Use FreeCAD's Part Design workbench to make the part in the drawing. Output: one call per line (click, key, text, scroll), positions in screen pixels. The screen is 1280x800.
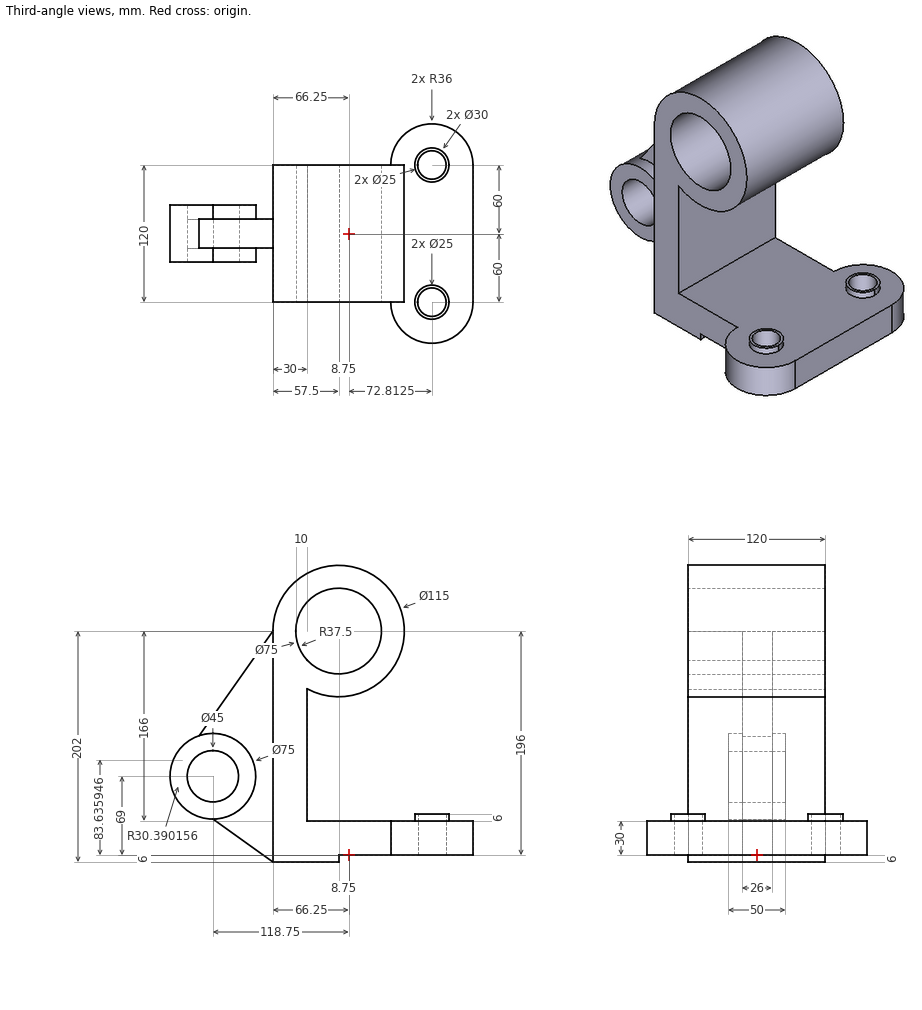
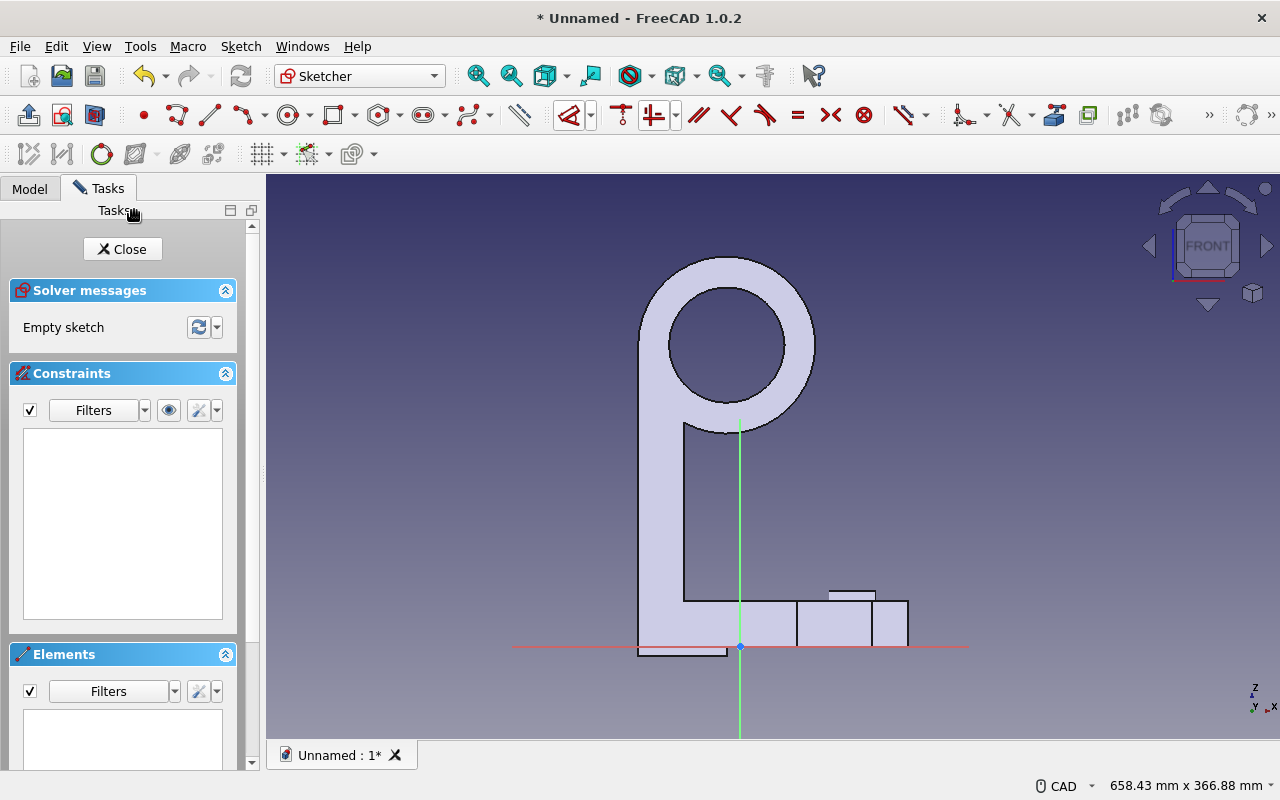
click(516, 518)
click(638, 345)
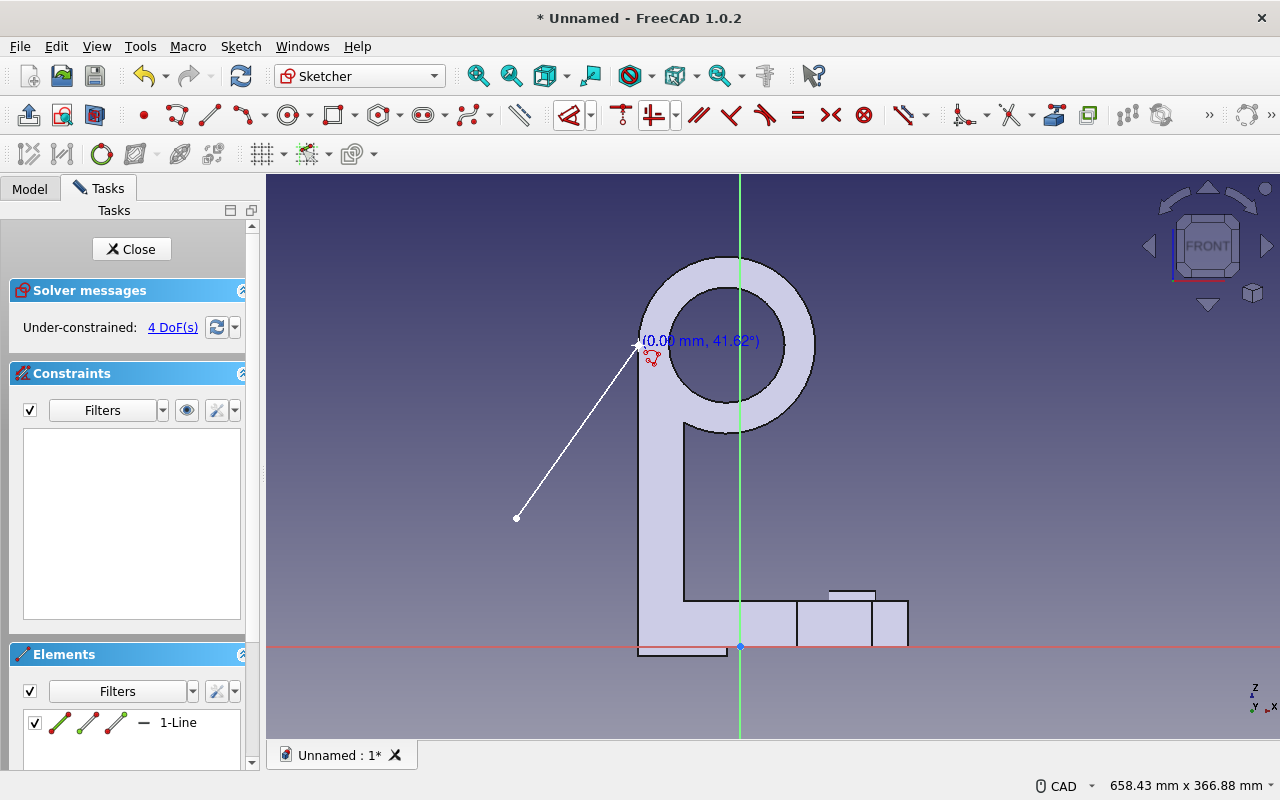
scroll(638, 656, up, 3)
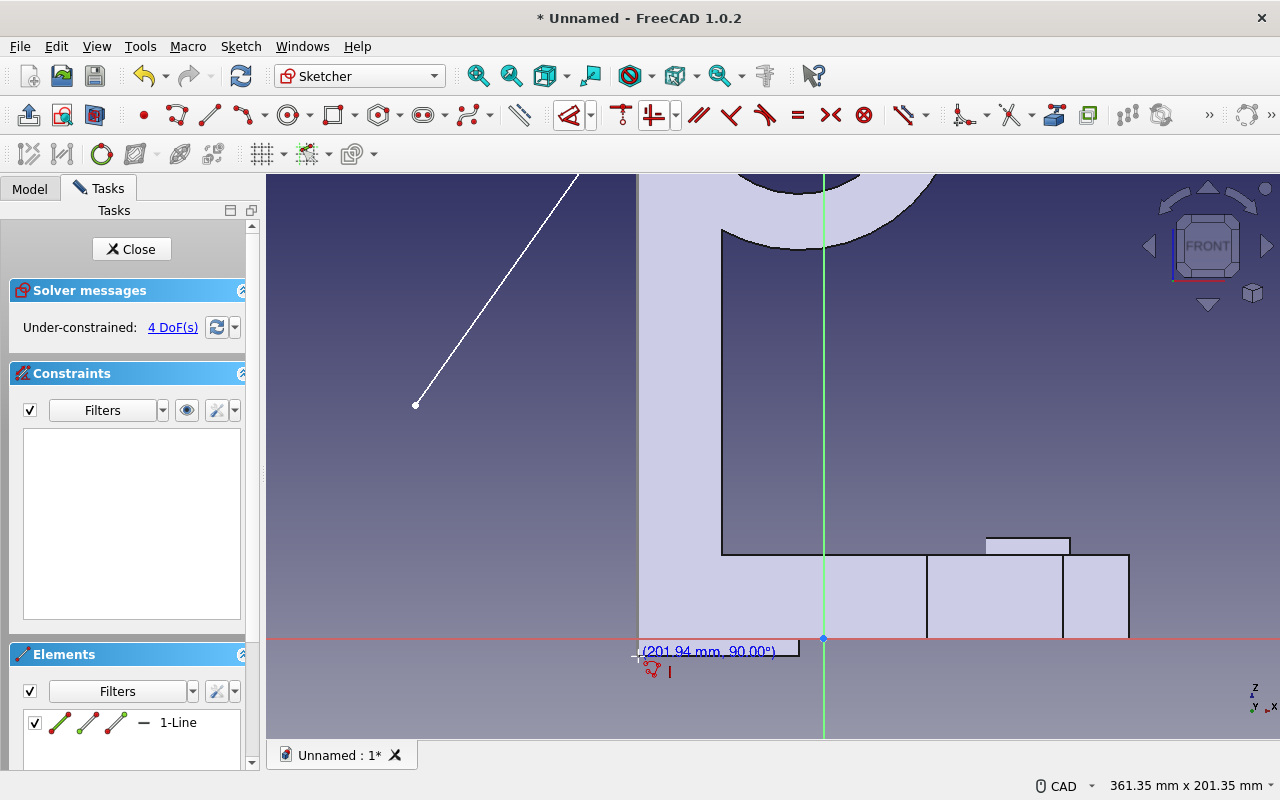
click(638, 656)
click(441, 514)
right_click(441, 514)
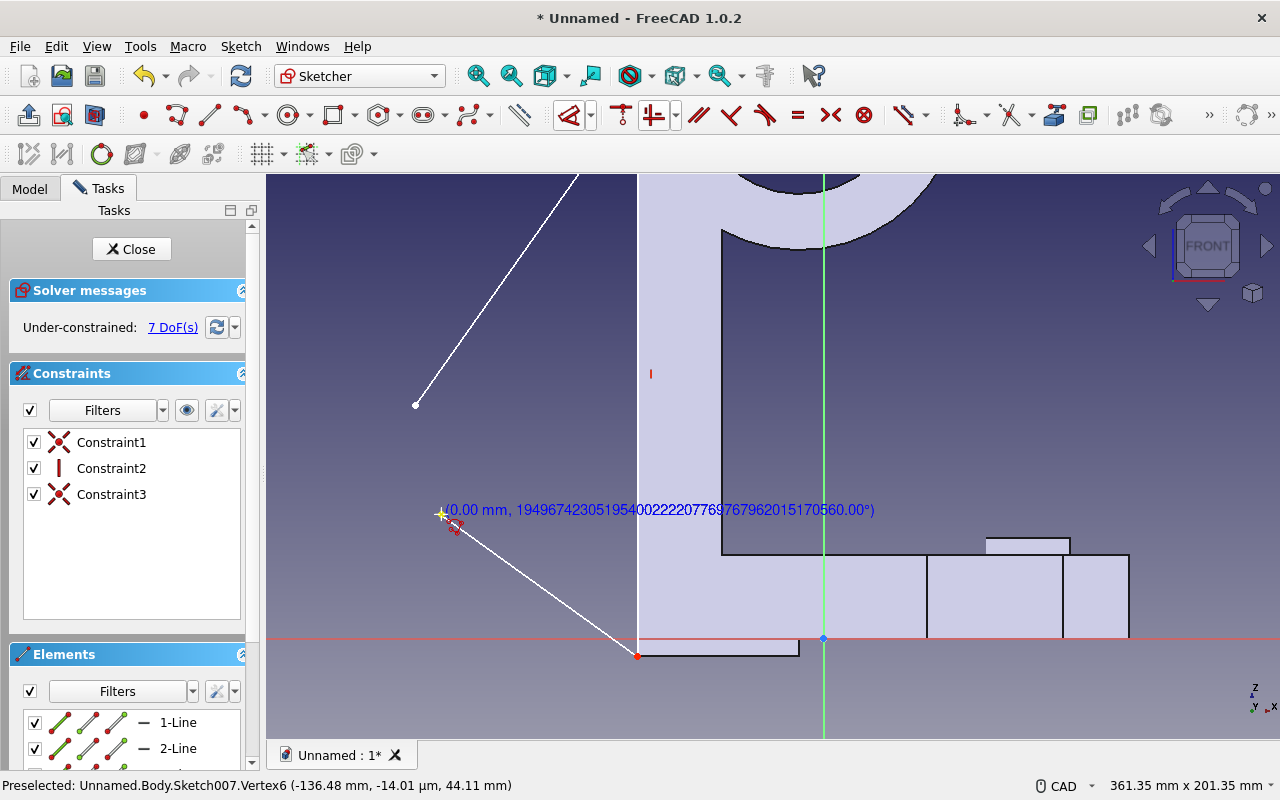
key(g)
key(3)
key(a)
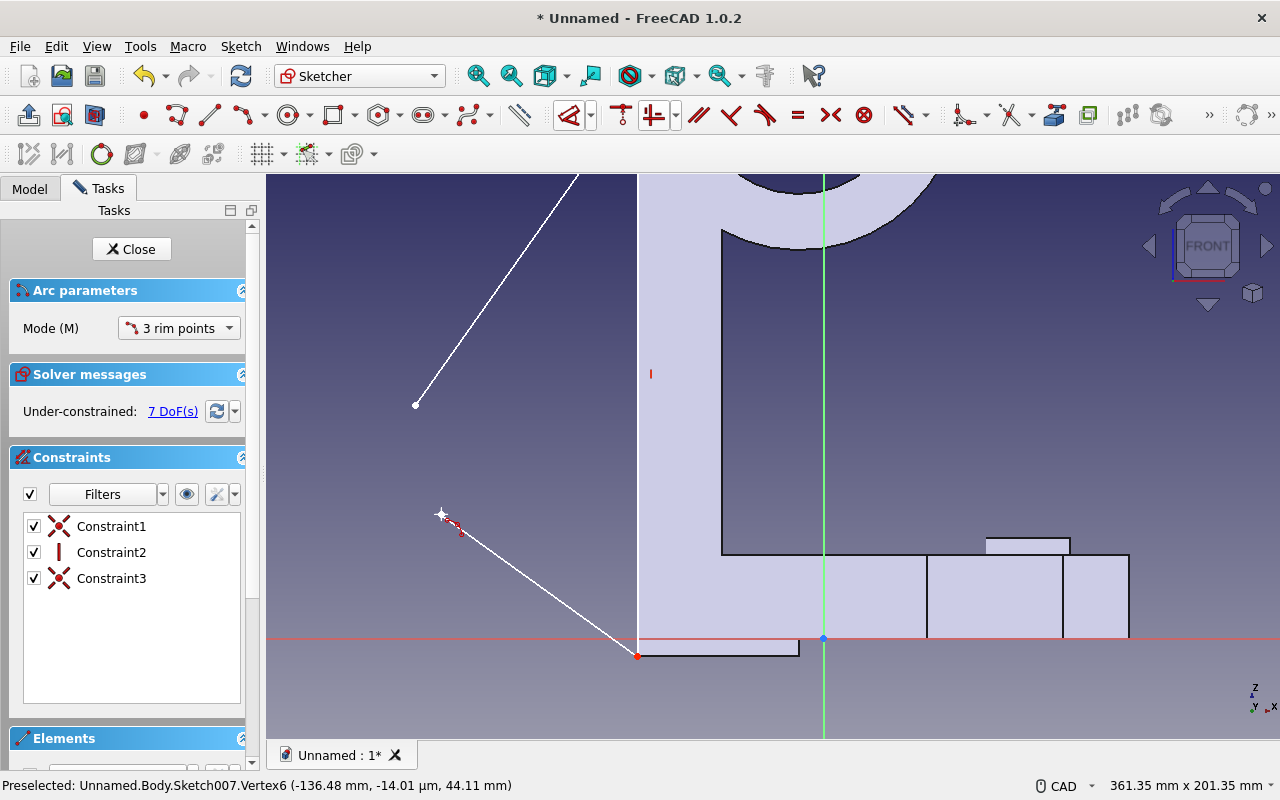
click(441, 515)
click(415, 406)
click(408, 464)
key(Escape)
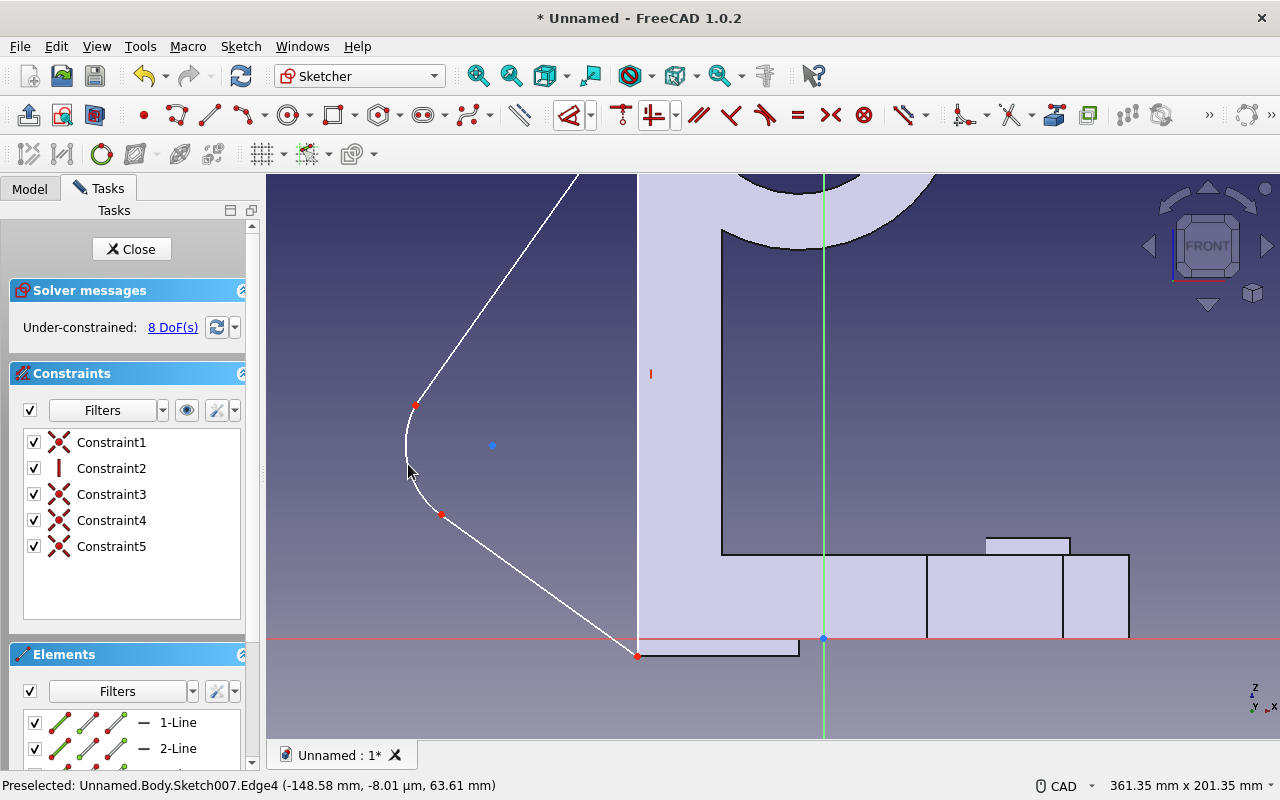
click(579, 614)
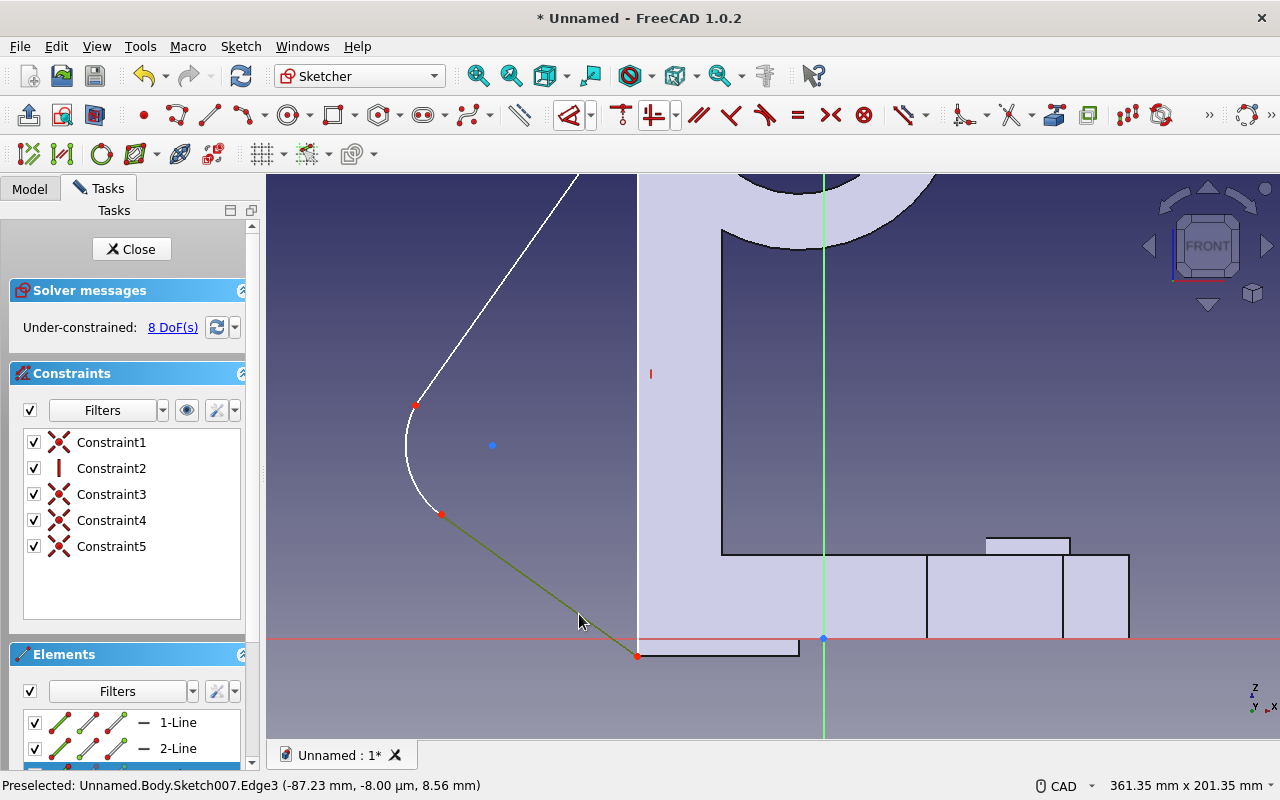
click(406, 441)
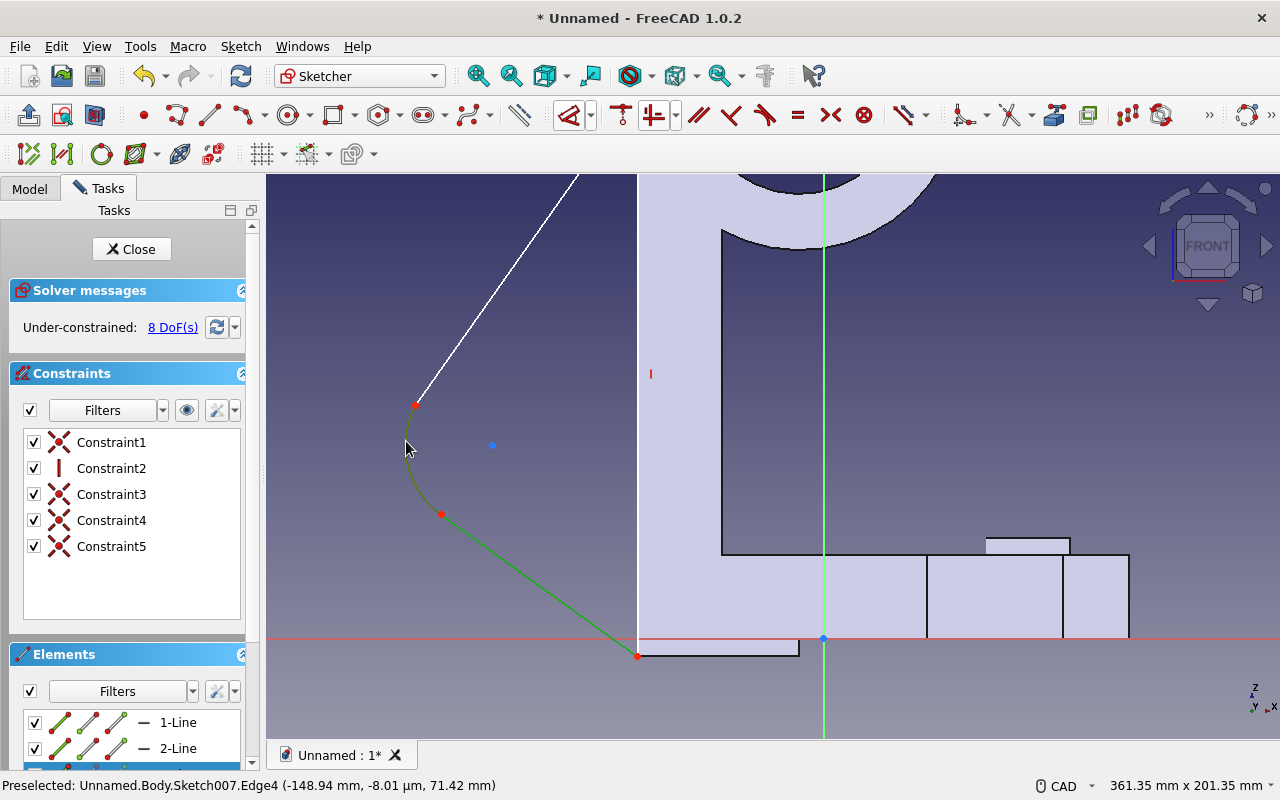
key(t)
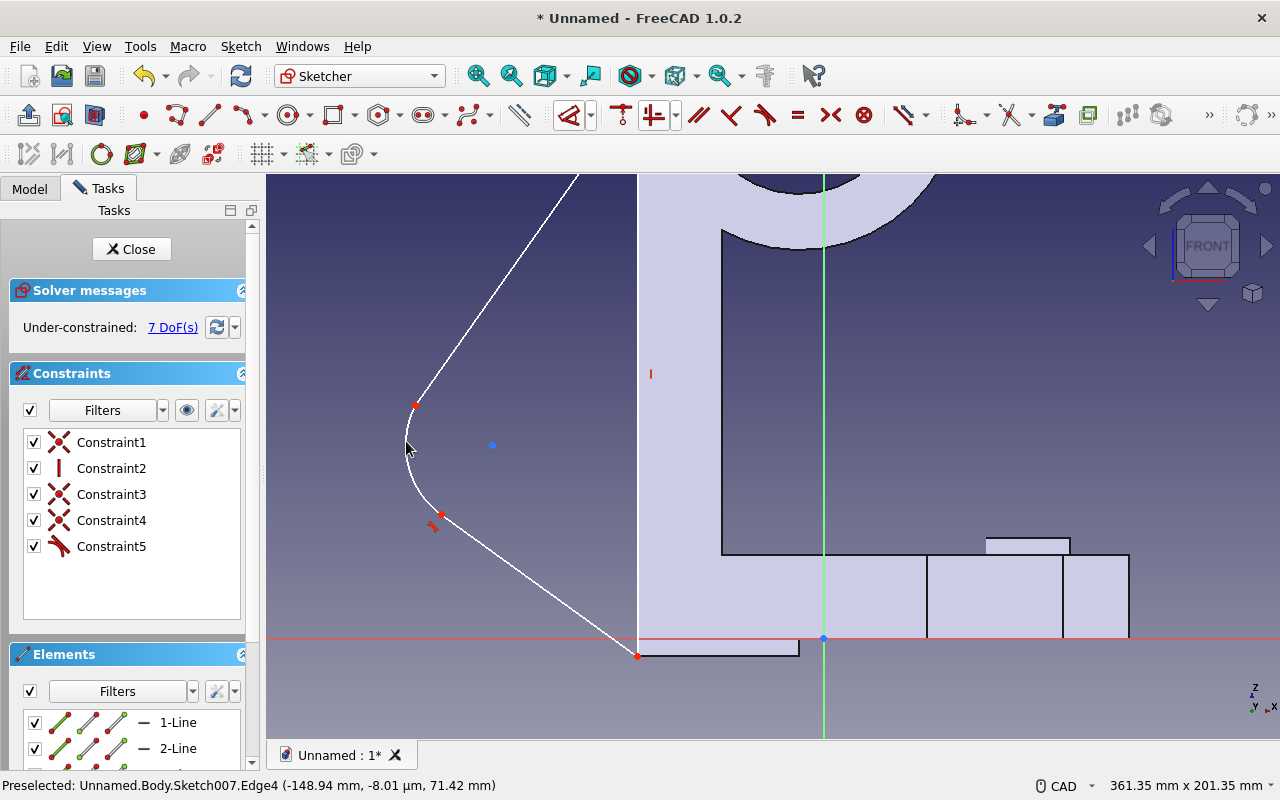
click(406, 441)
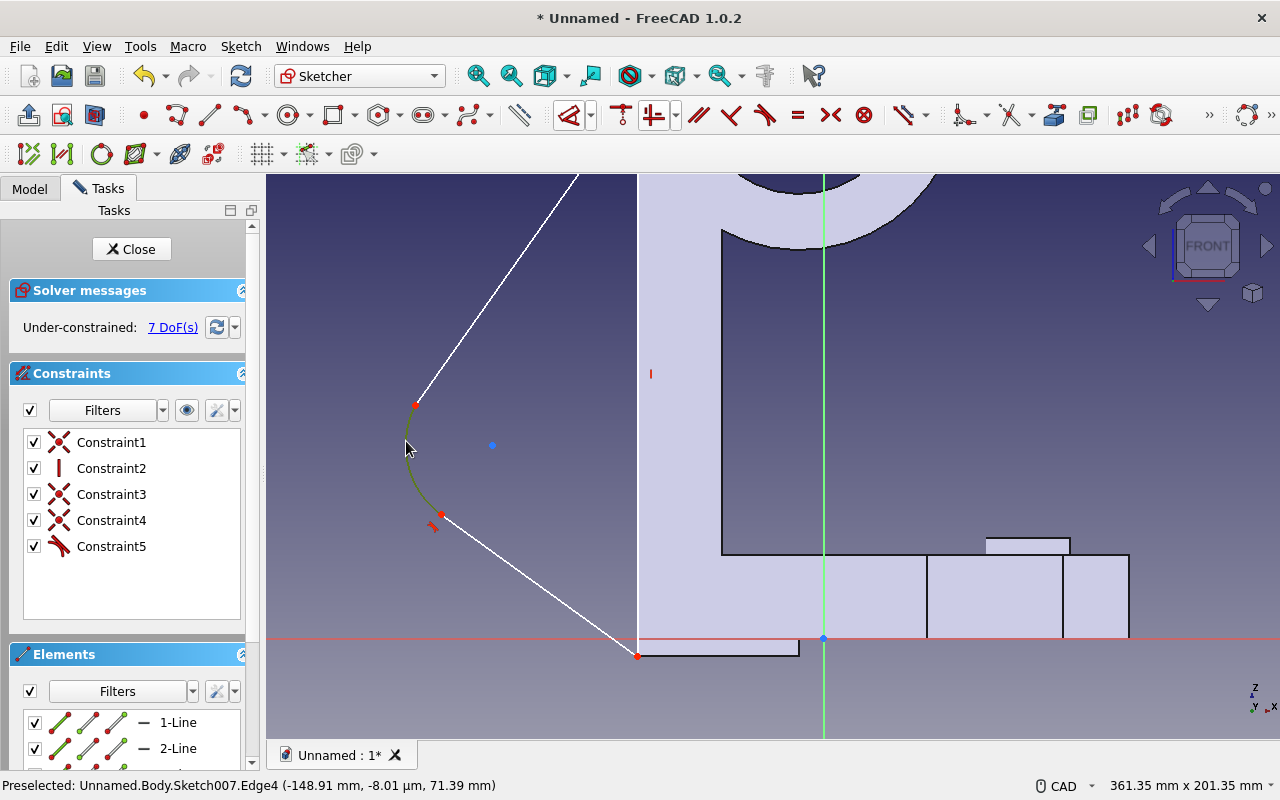
click(590, 116)